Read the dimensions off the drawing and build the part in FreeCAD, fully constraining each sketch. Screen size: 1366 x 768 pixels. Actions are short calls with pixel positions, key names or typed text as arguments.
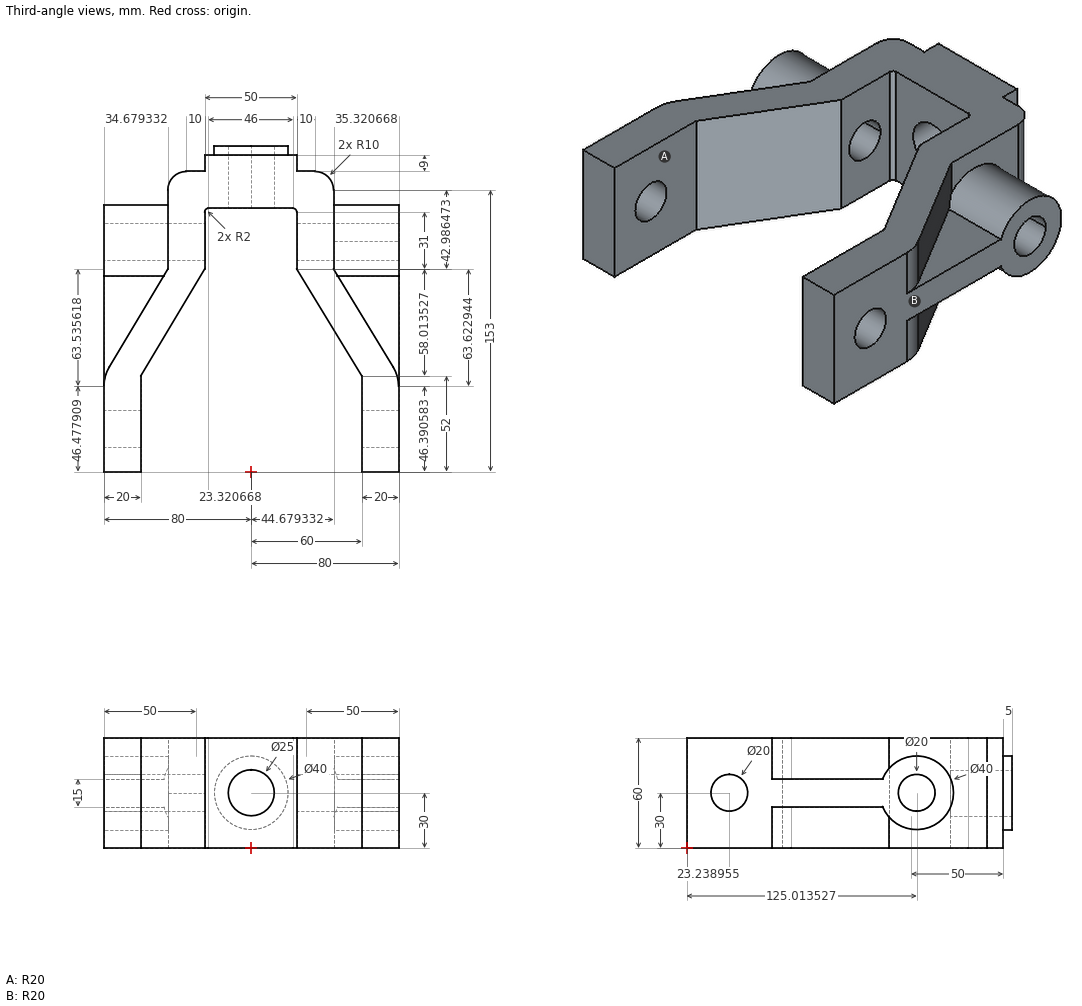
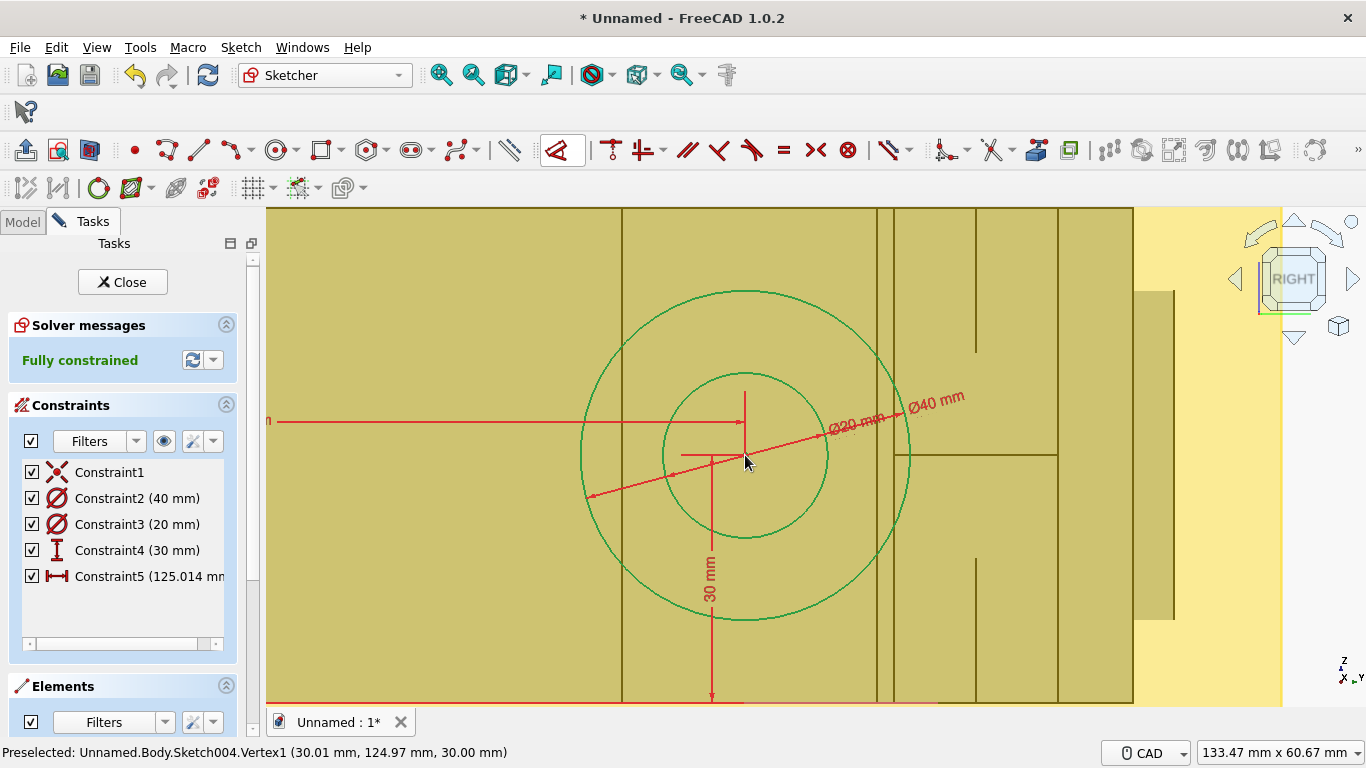
click(123, 282)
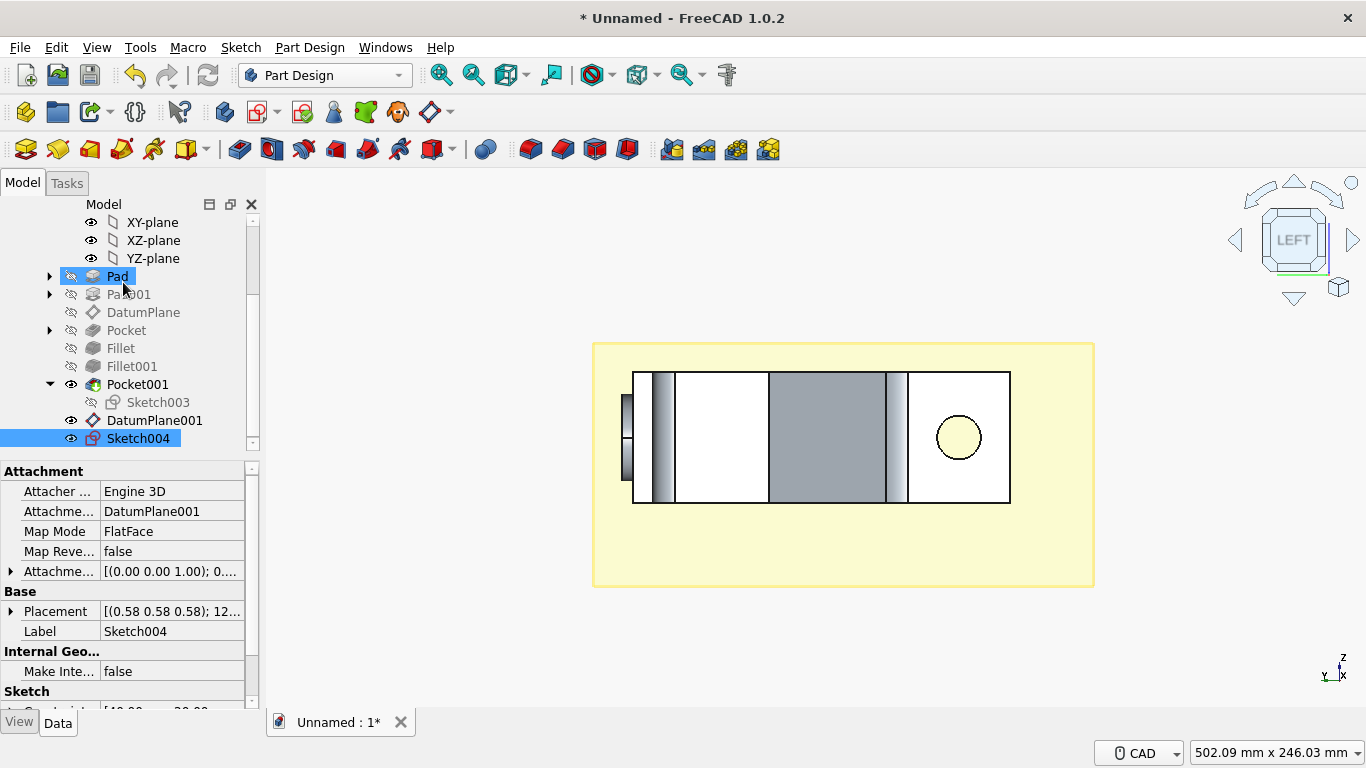
click(26, 150)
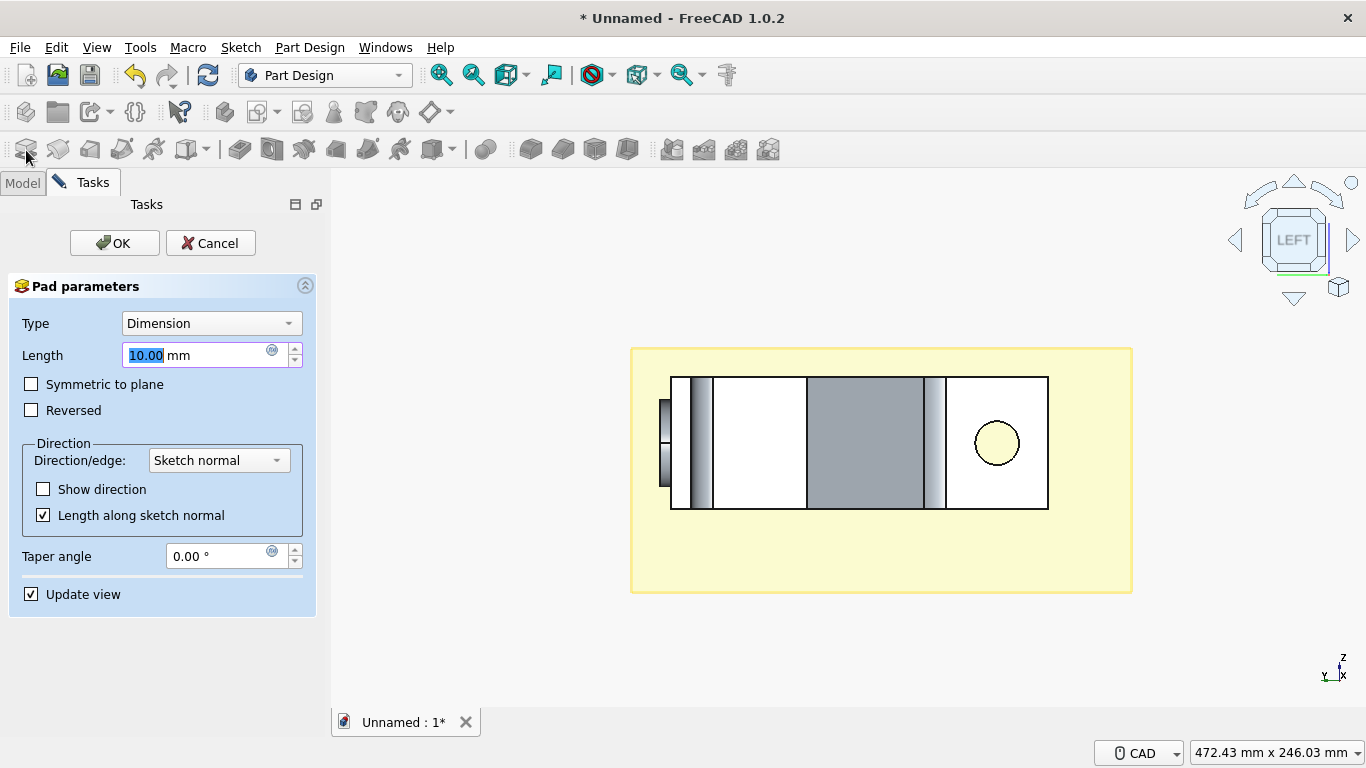
text(50)
key(Tab)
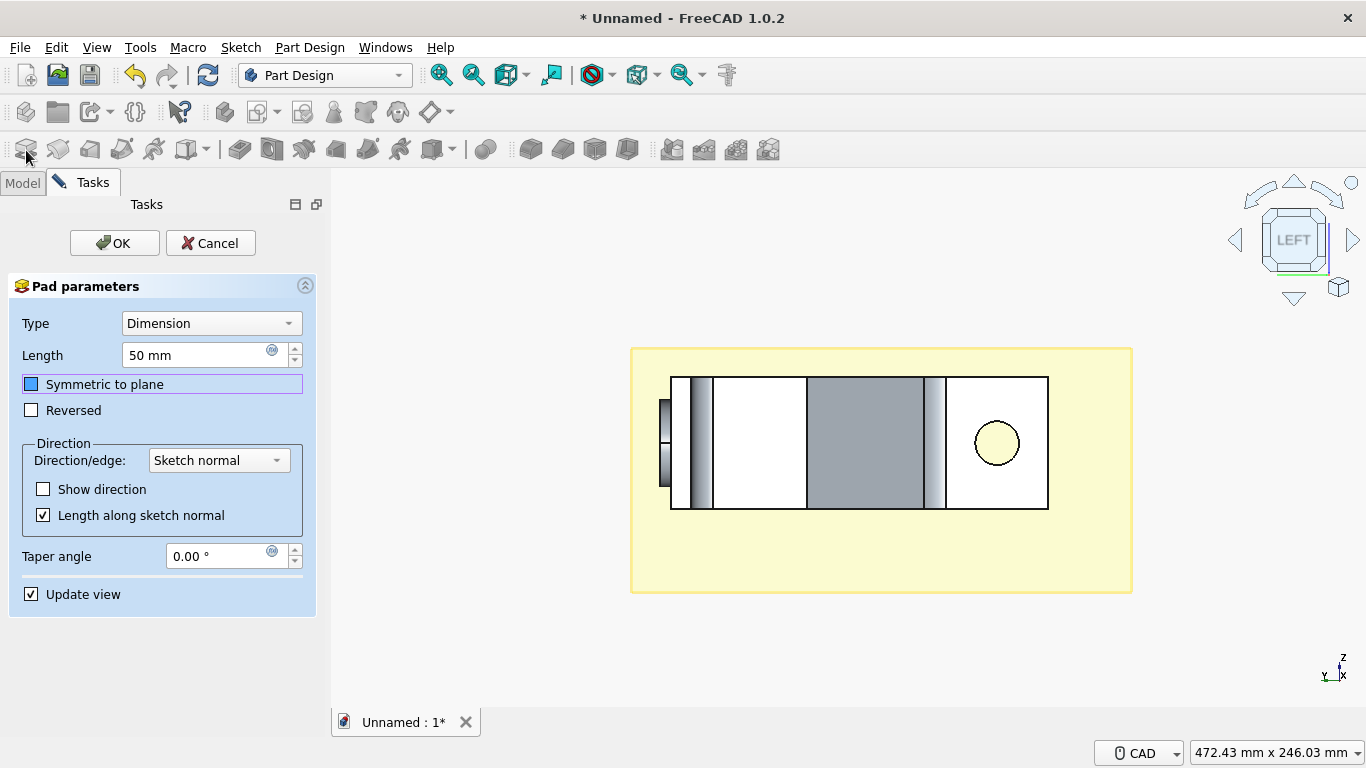
click(115, 243)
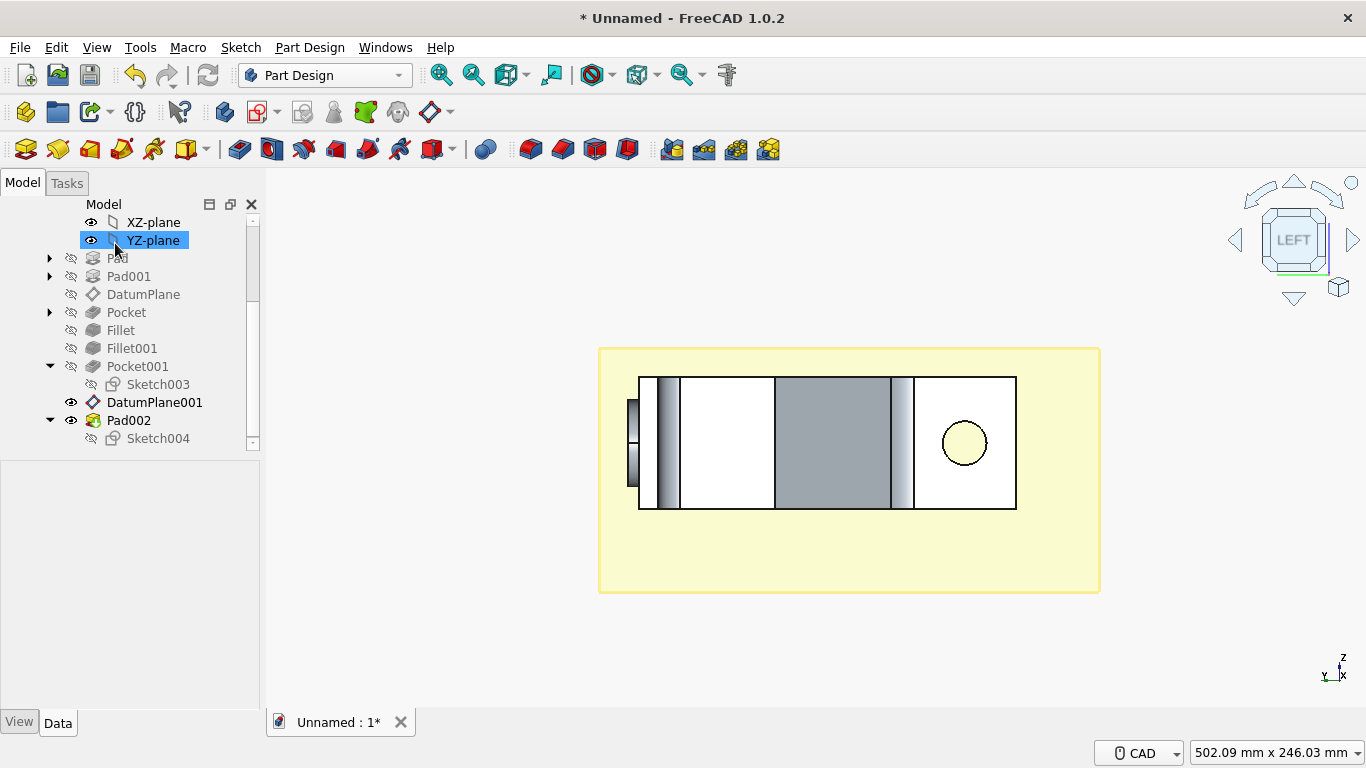
click(116, 402)
key(space)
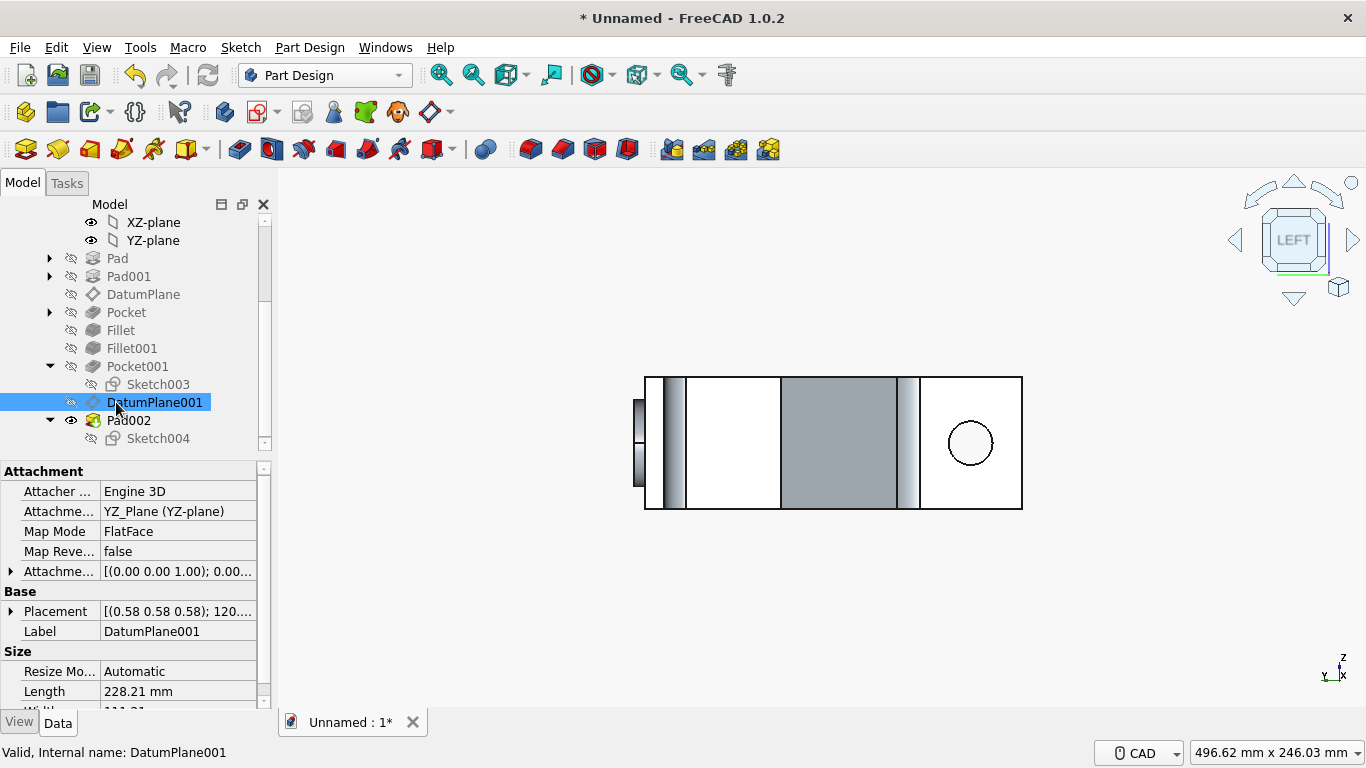
key(v)
key(f)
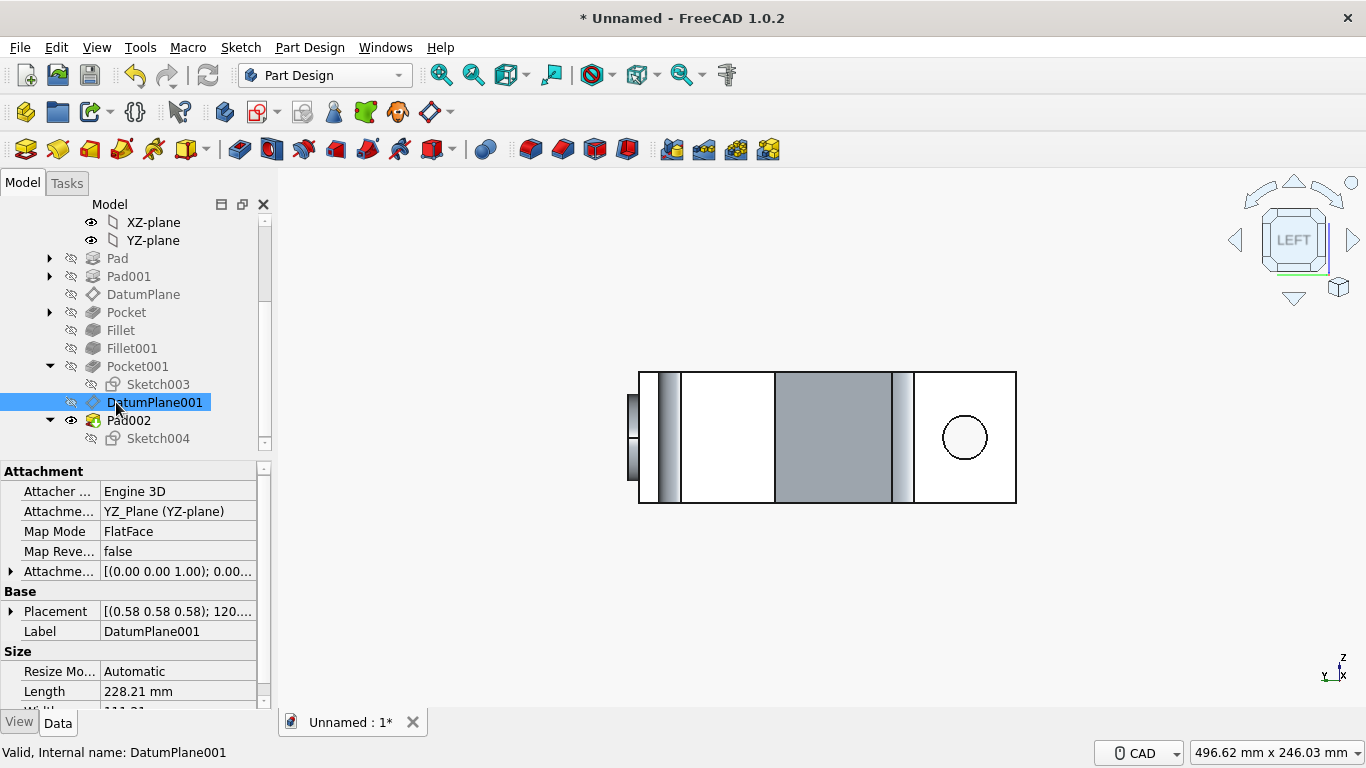
click(936, 399)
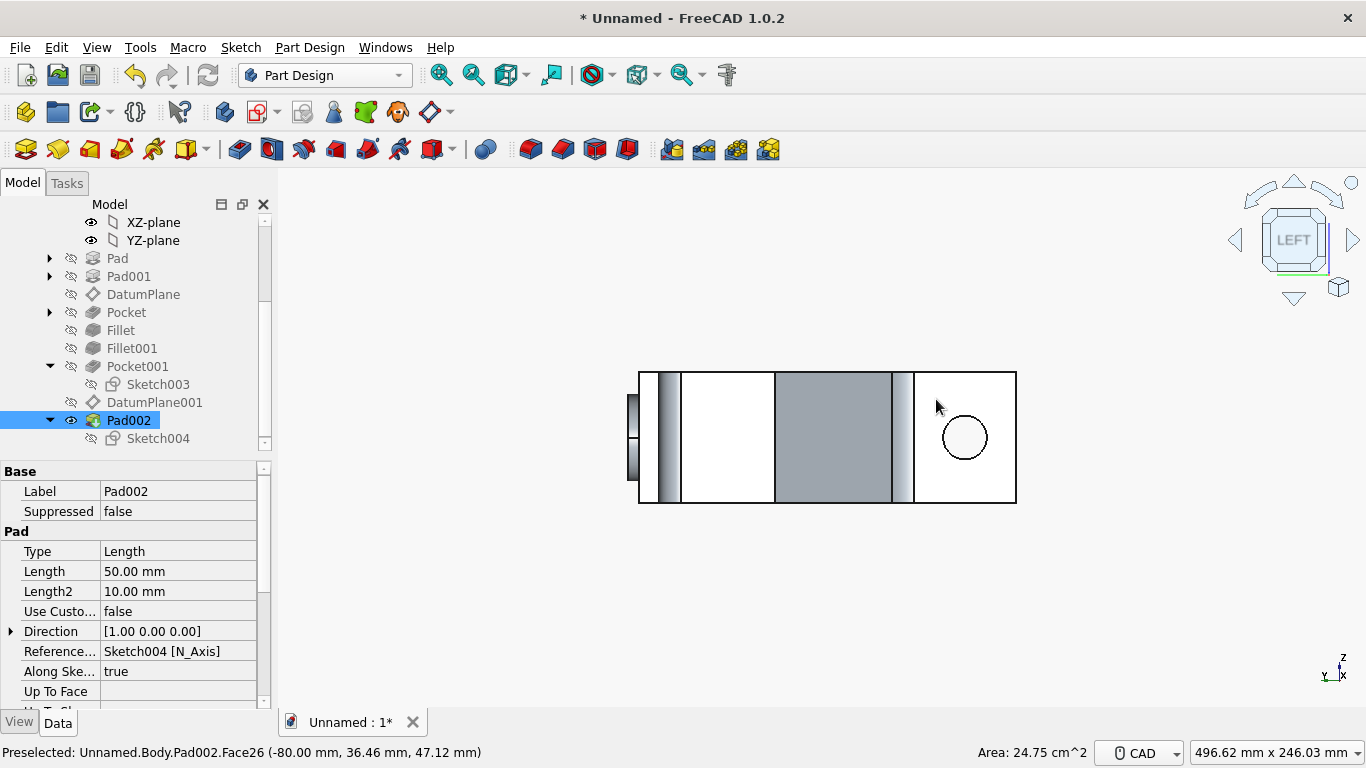
click(258, 112)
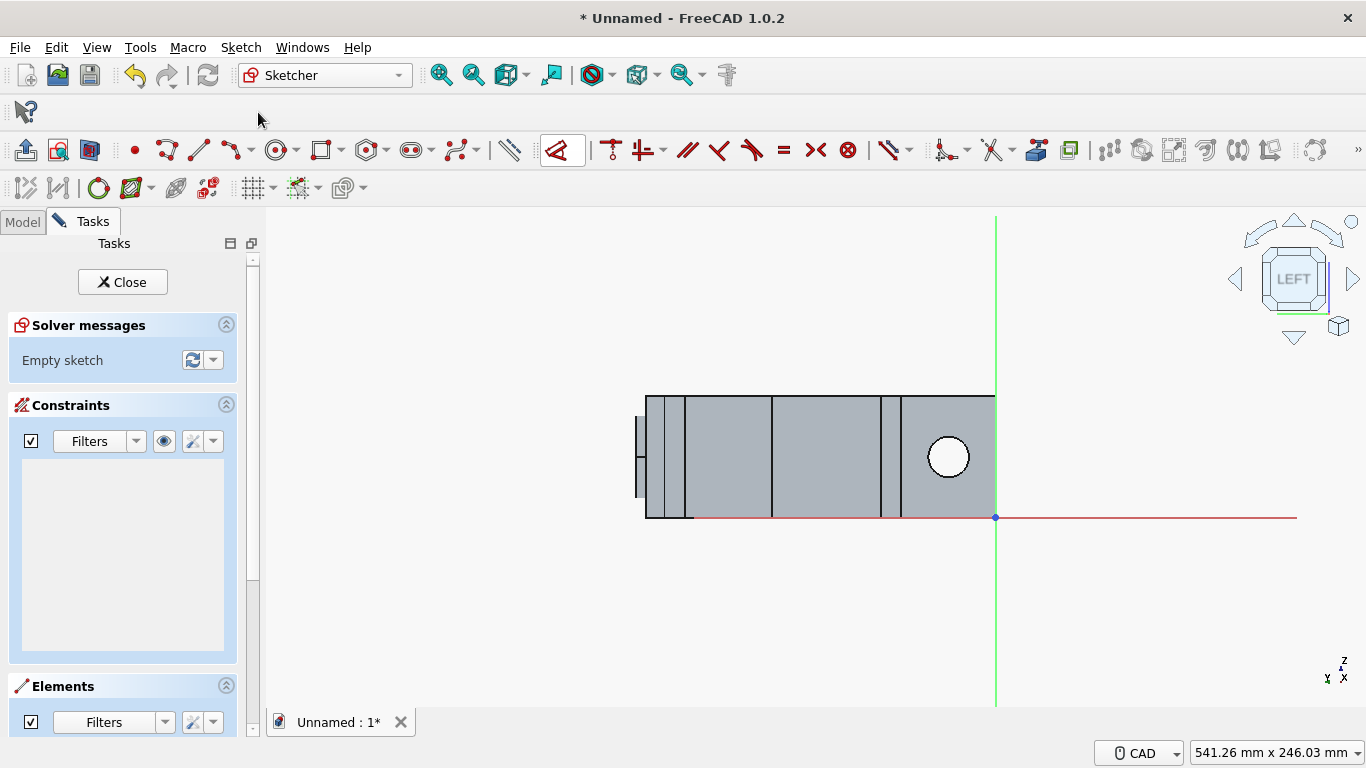
scroll(740, 457, up, 7)